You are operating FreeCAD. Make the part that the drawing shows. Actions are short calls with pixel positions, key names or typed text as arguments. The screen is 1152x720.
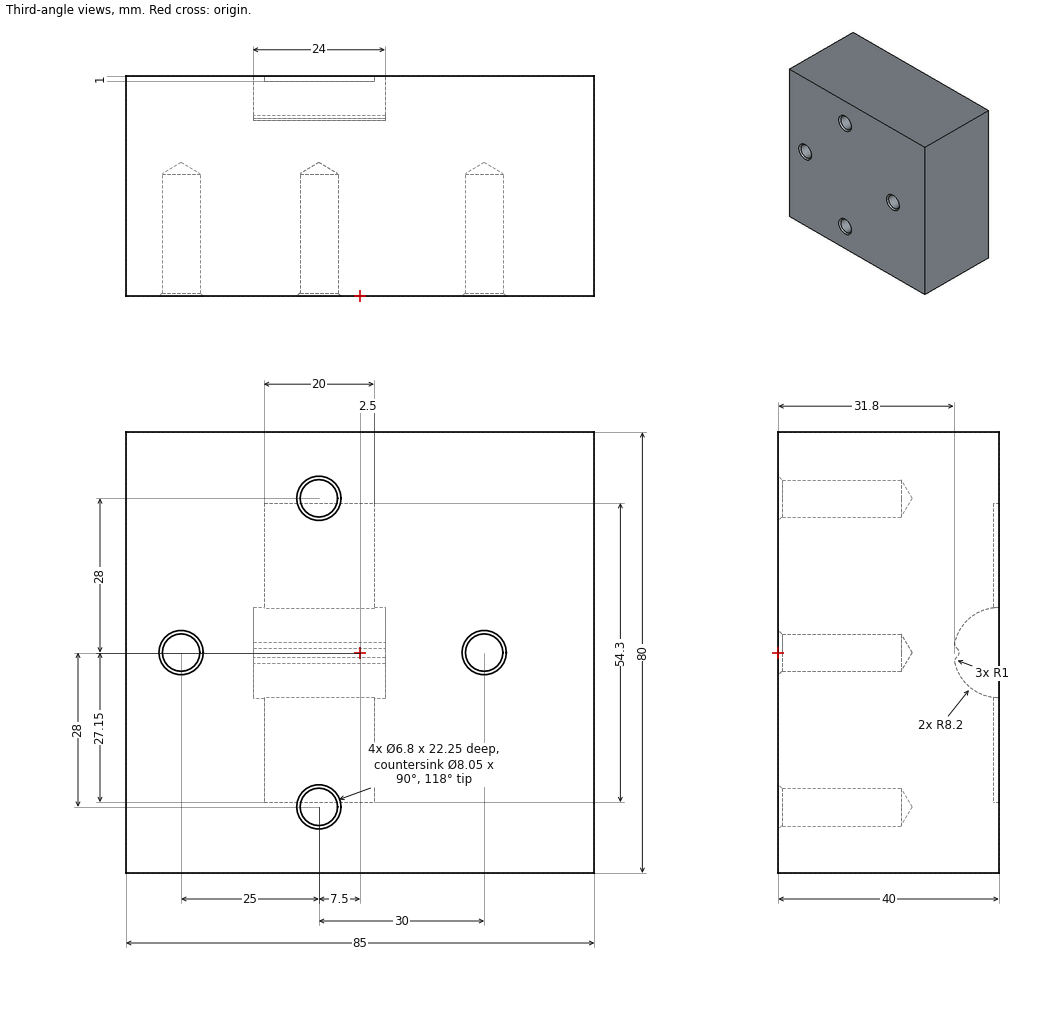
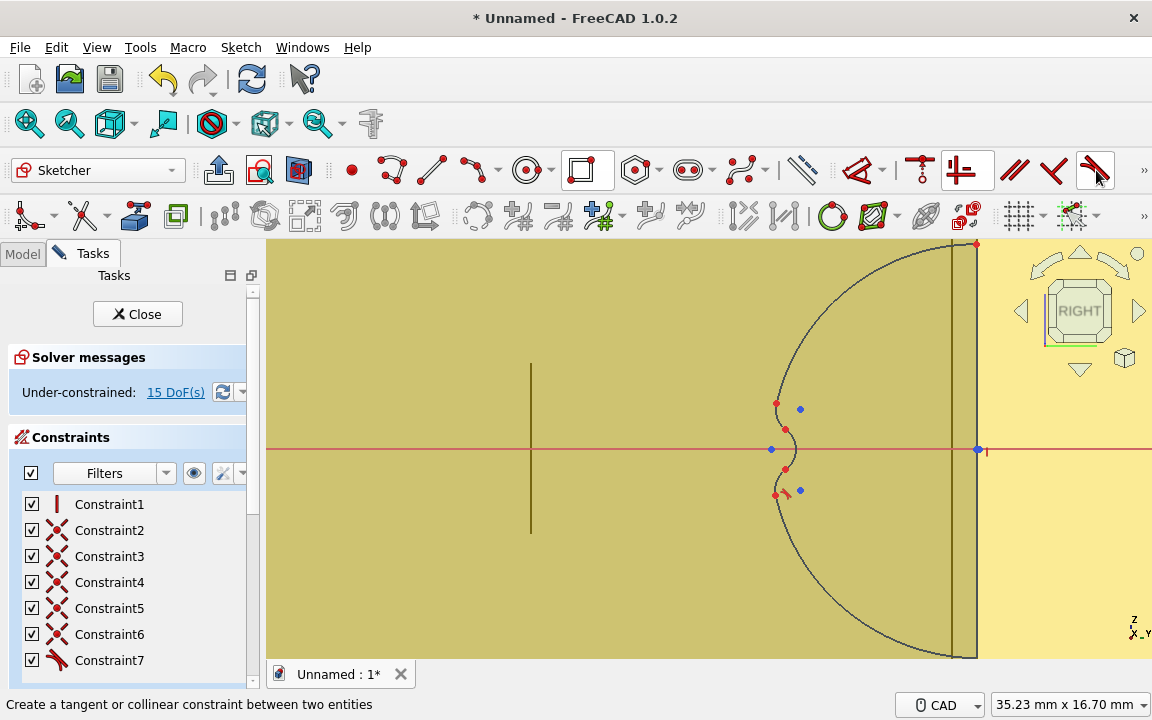
click(777, 481)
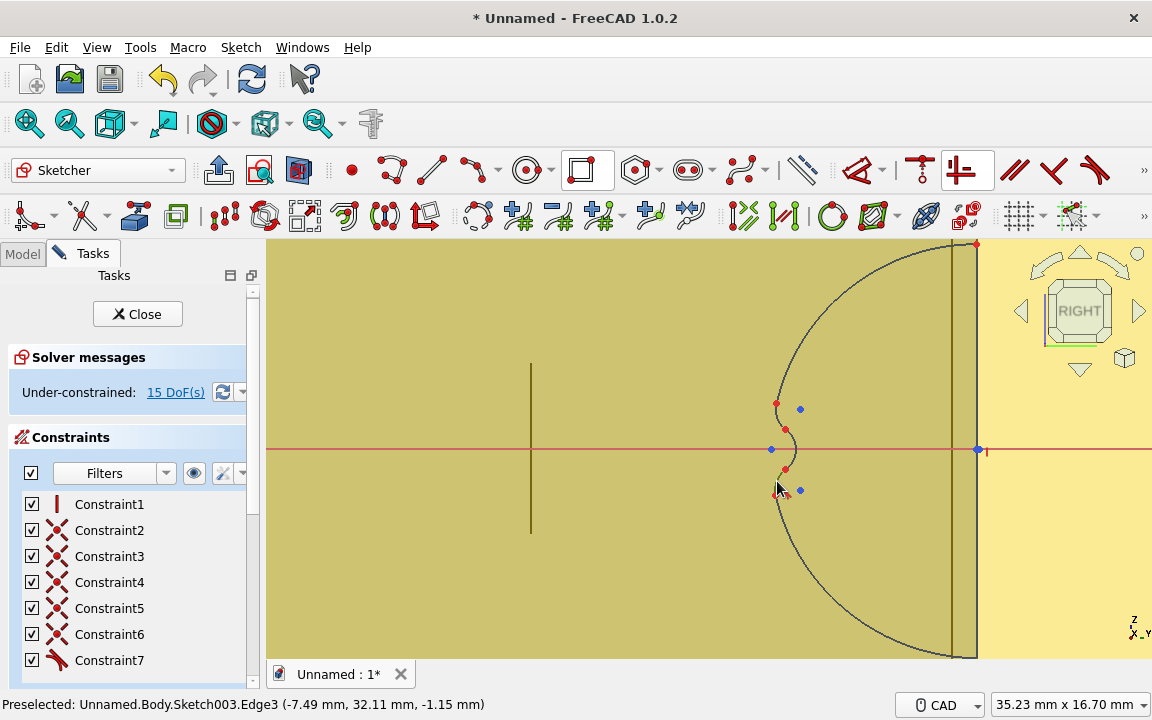
scroll(794, 459, up, 2)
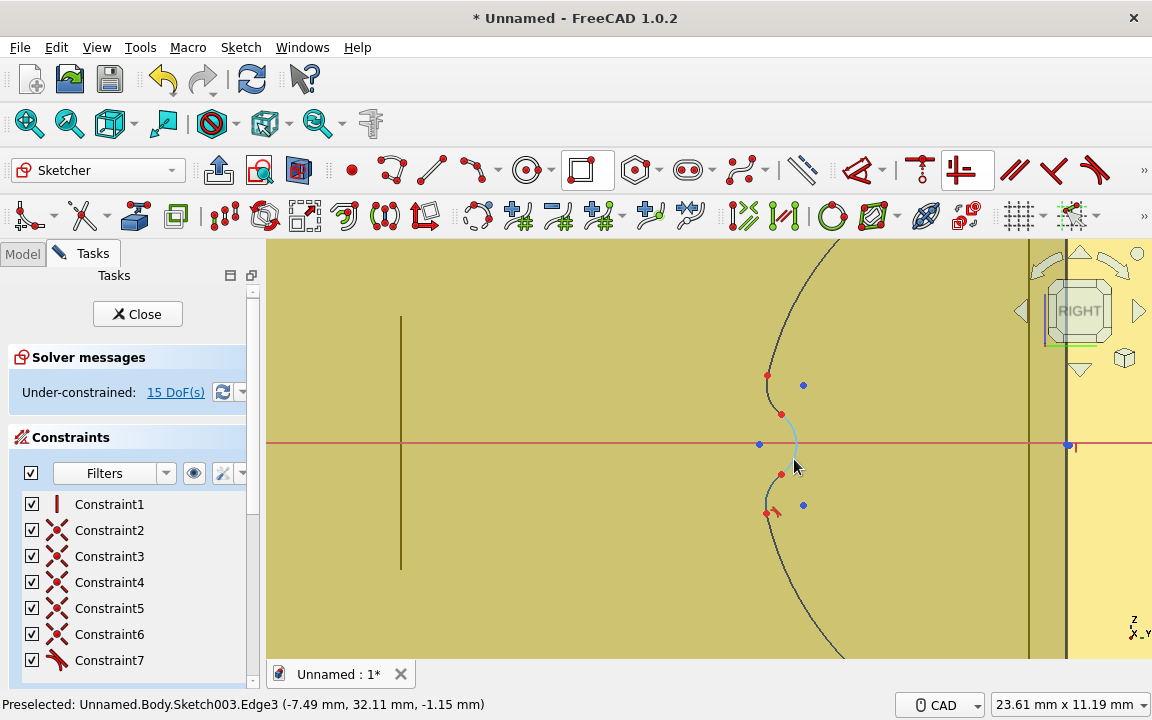
click(794, 458)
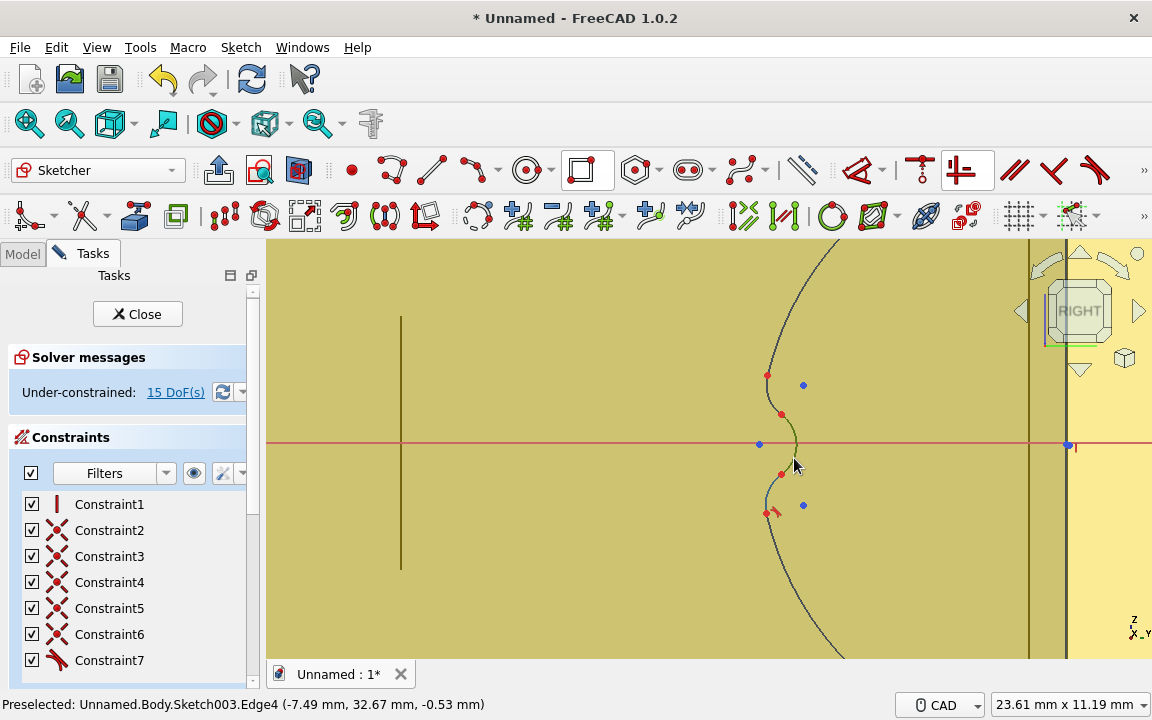
click(1096, 170)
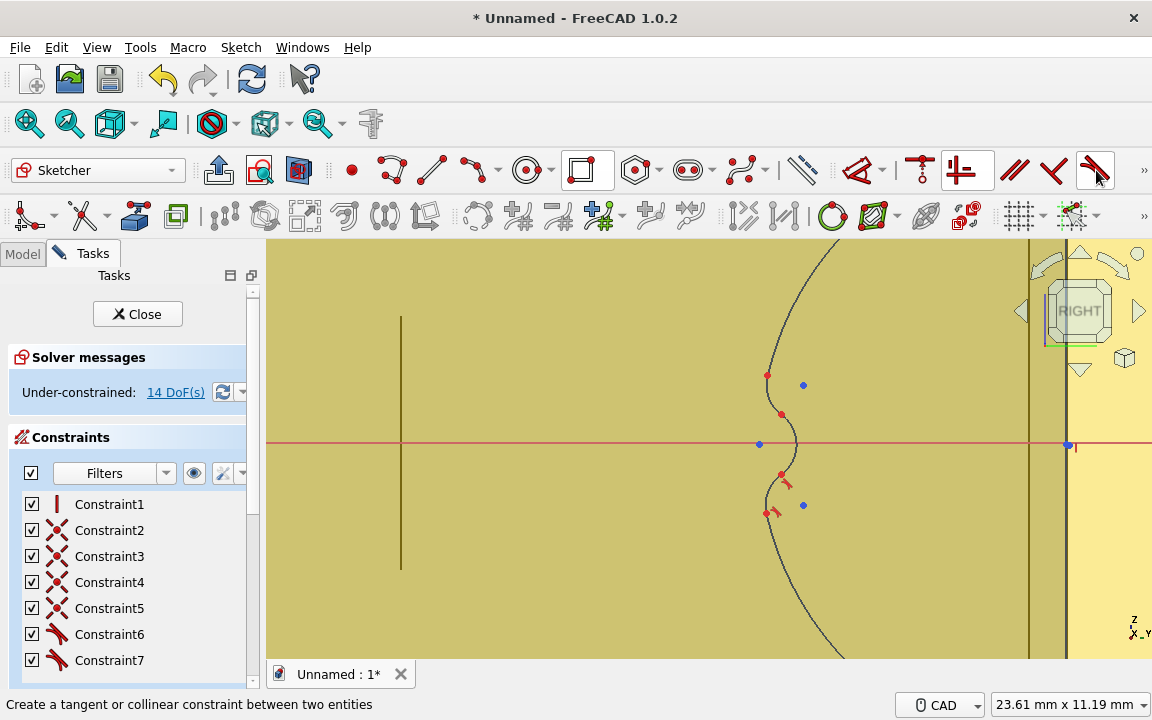
click(794, 458)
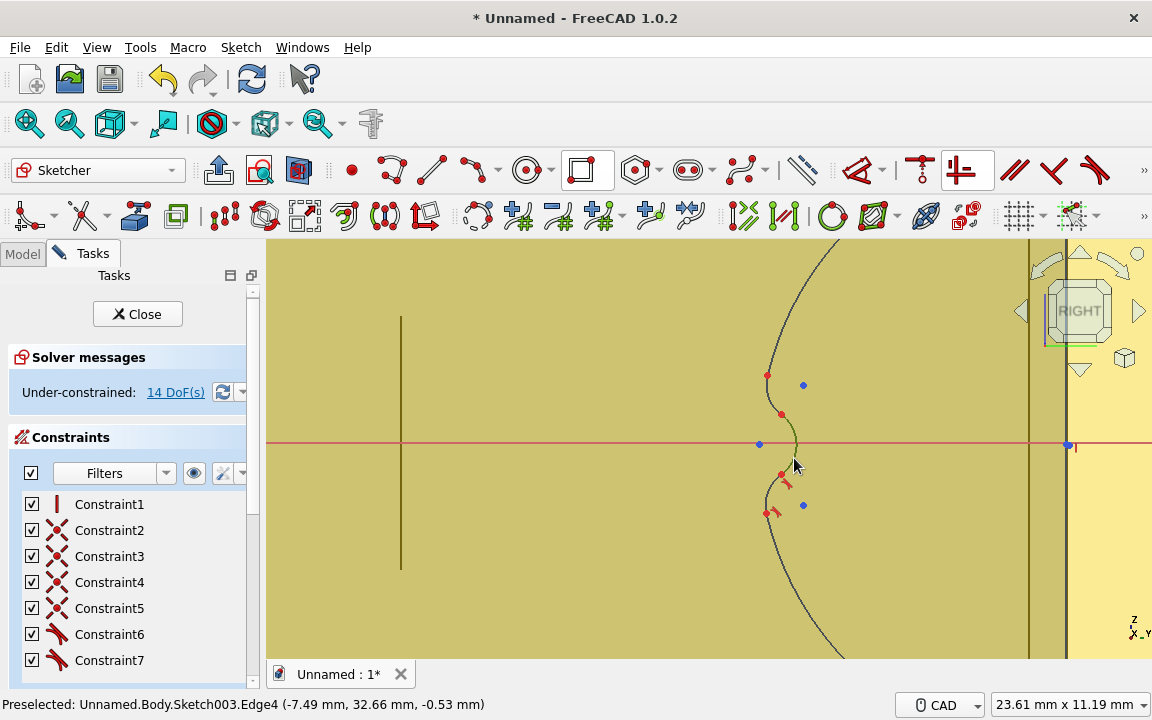
click(767, 389)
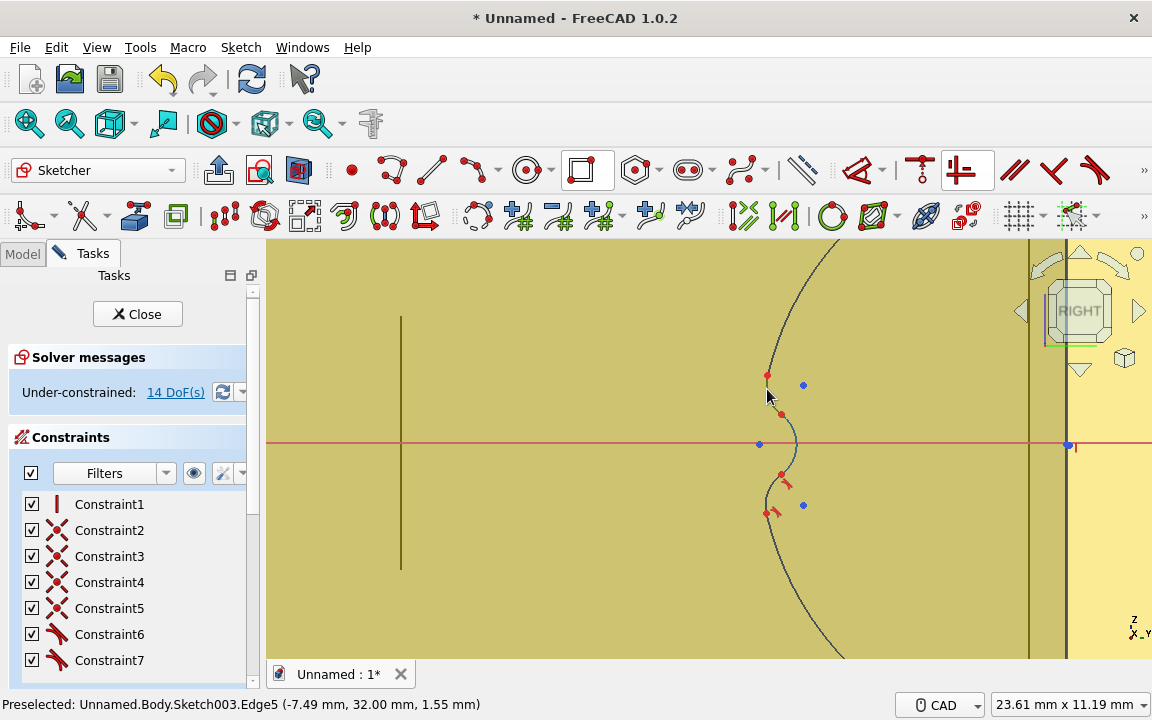
click(1096, 170)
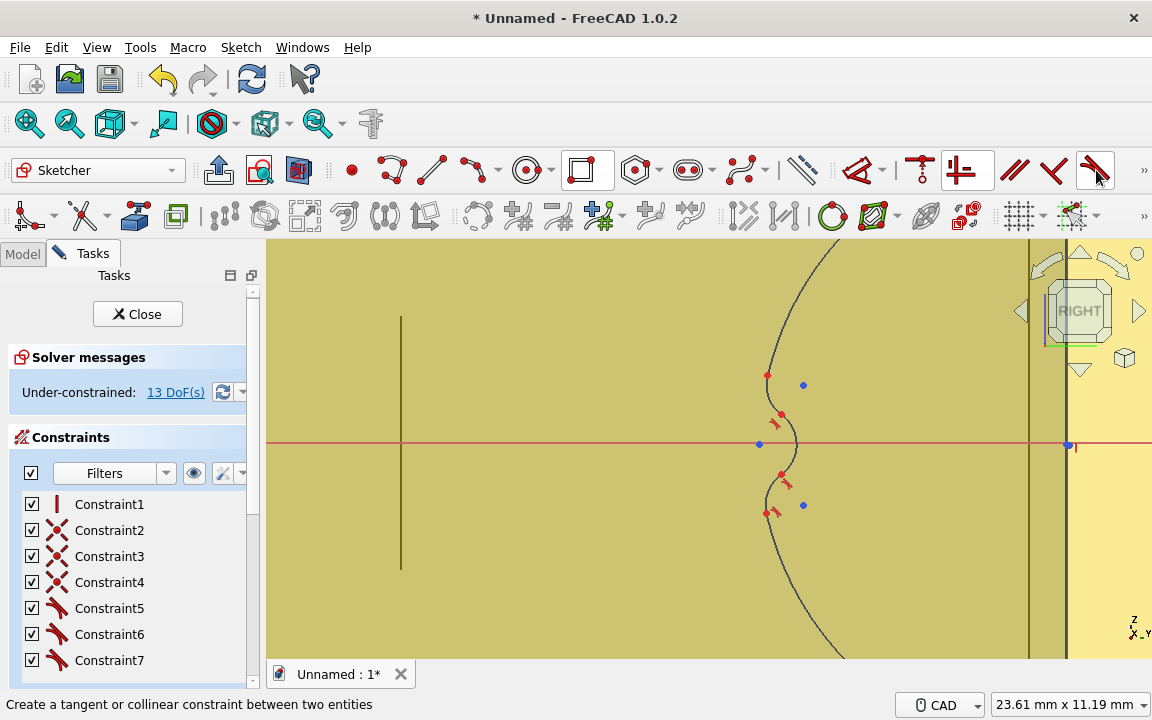
click(767, 389)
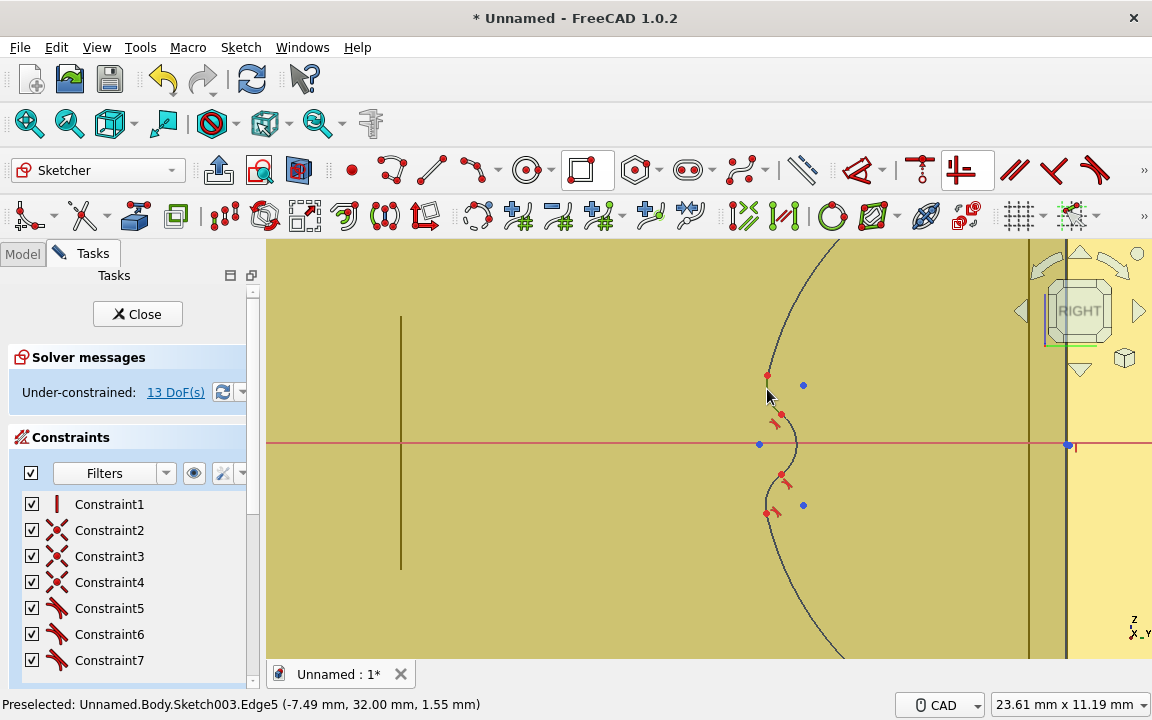
click(797, 299)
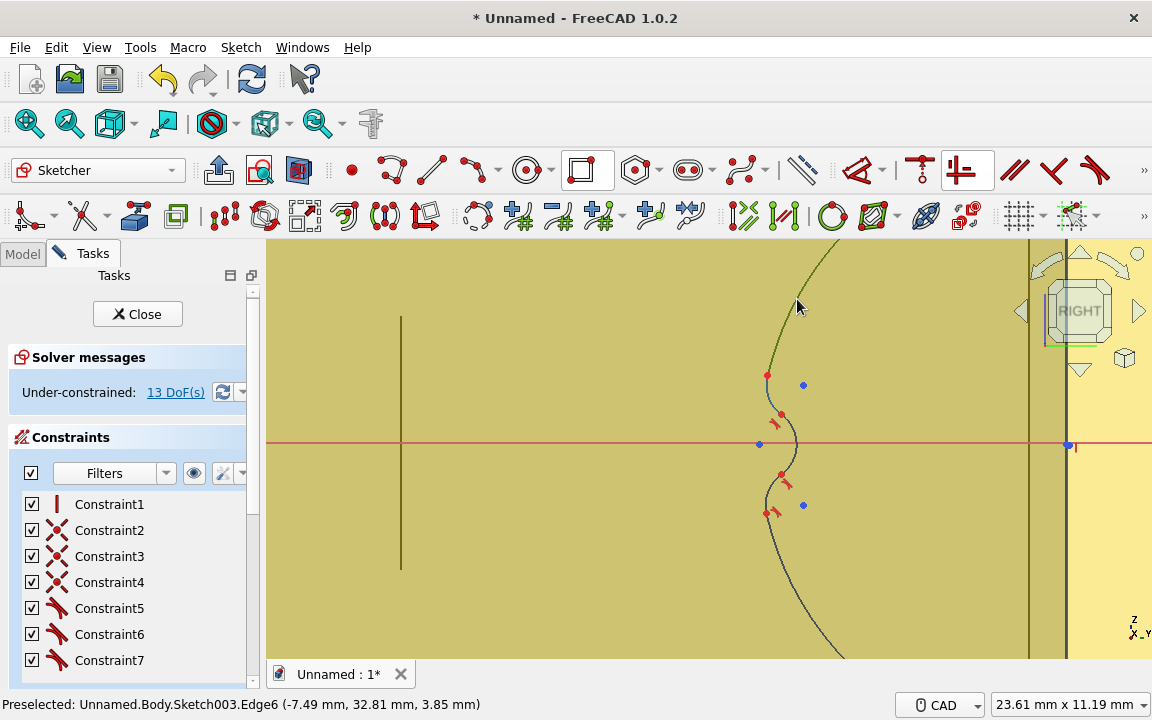
click(1096, 170)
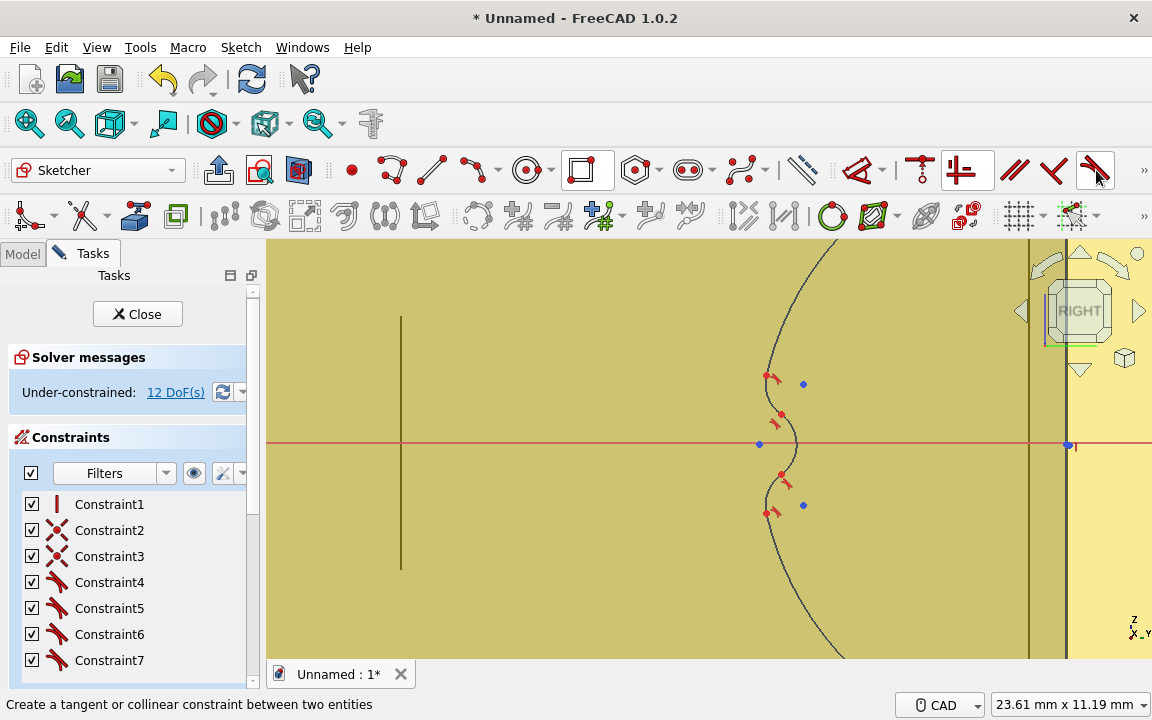
click(817, 627)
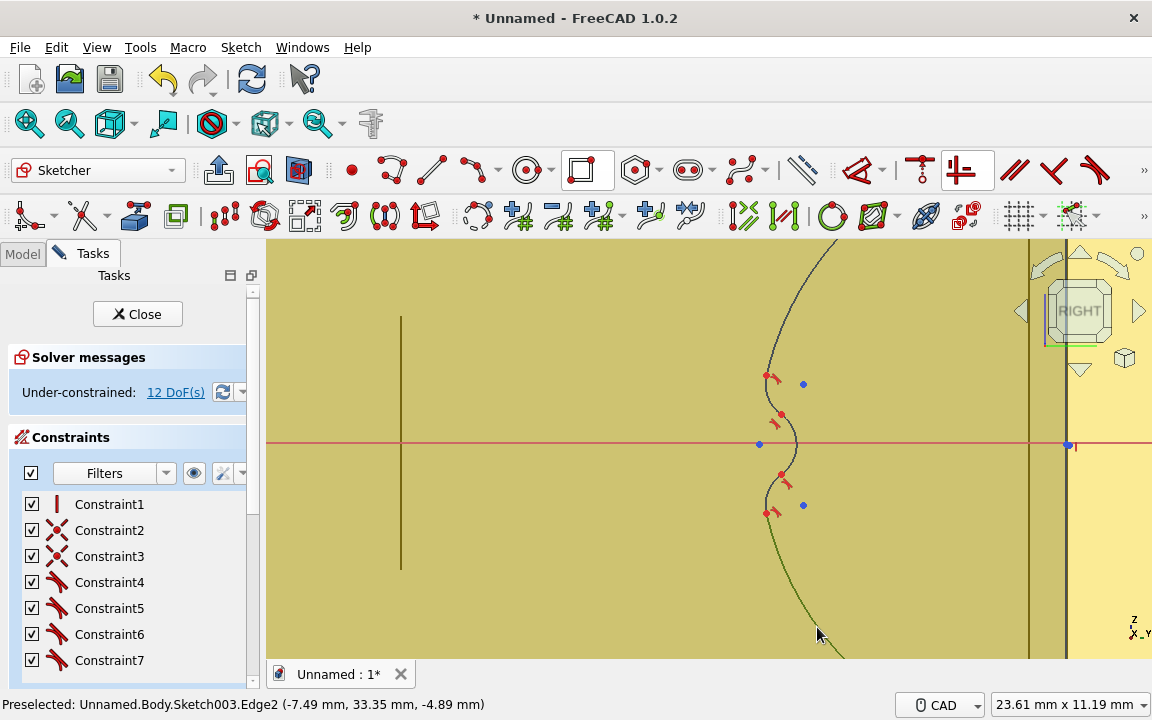
click(796, 298)